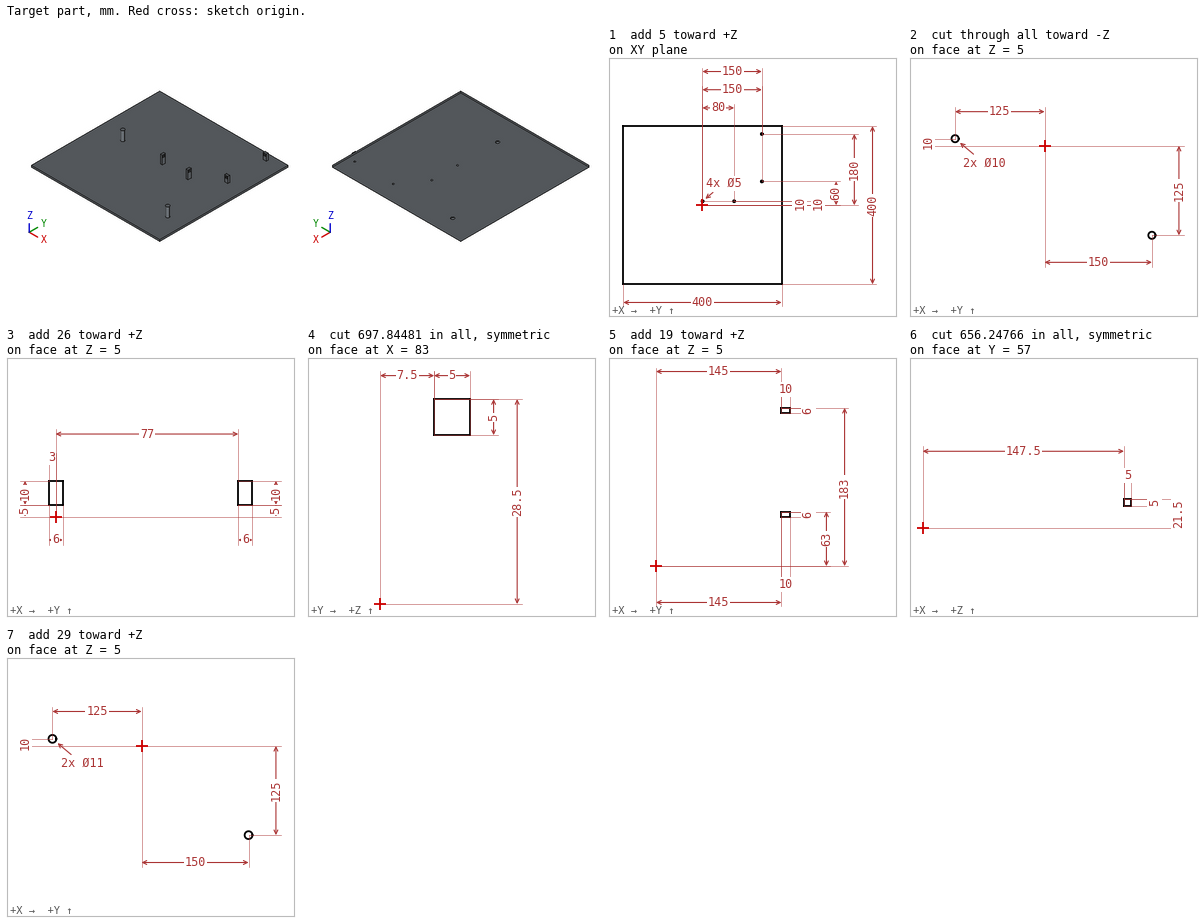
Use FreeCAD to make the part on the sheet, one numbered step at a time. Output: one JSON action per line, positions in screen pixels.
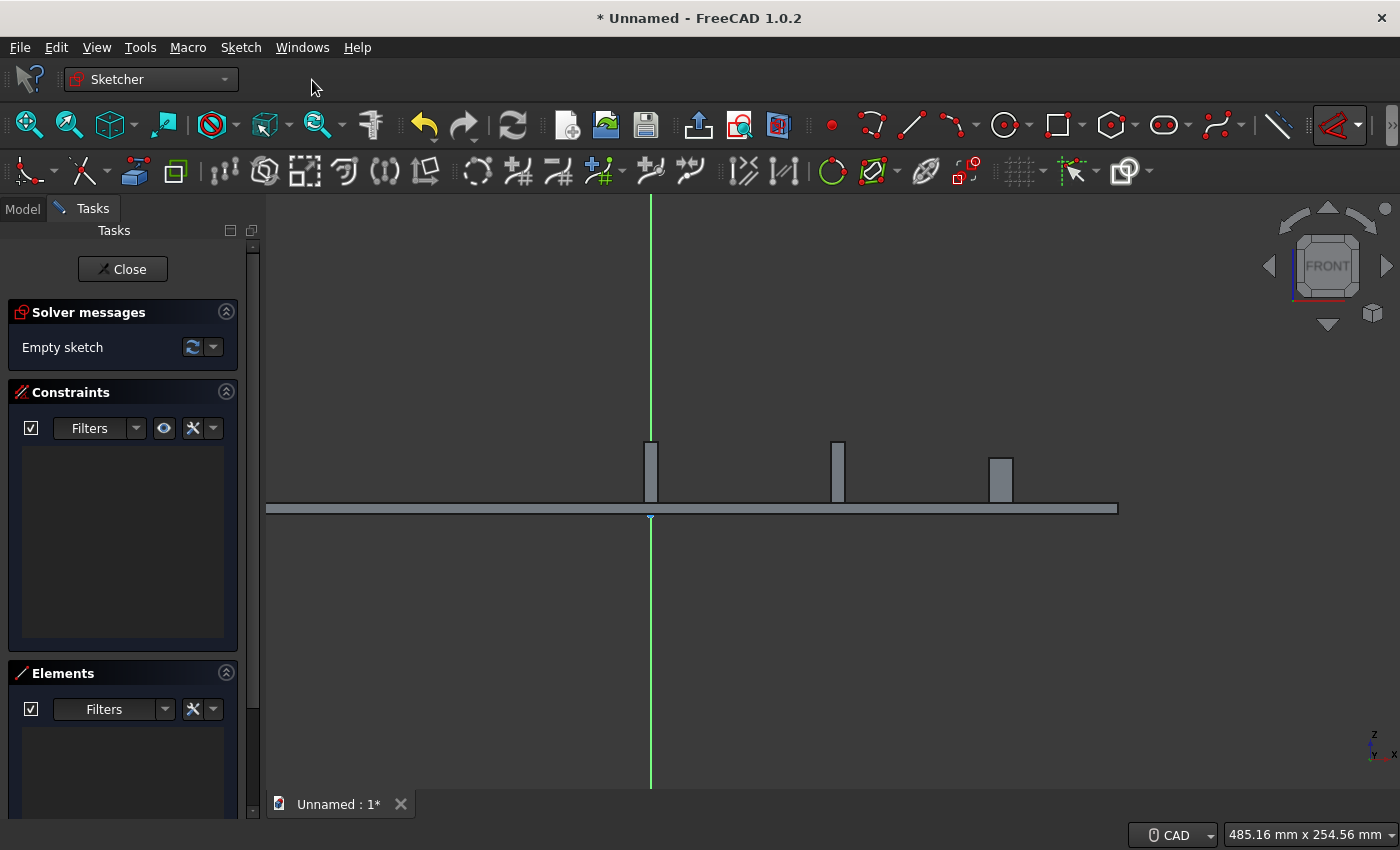
{"action": "scroll", "coordinate": [1014, 469], "scroll_direction": "up", "scroll_amount": 15}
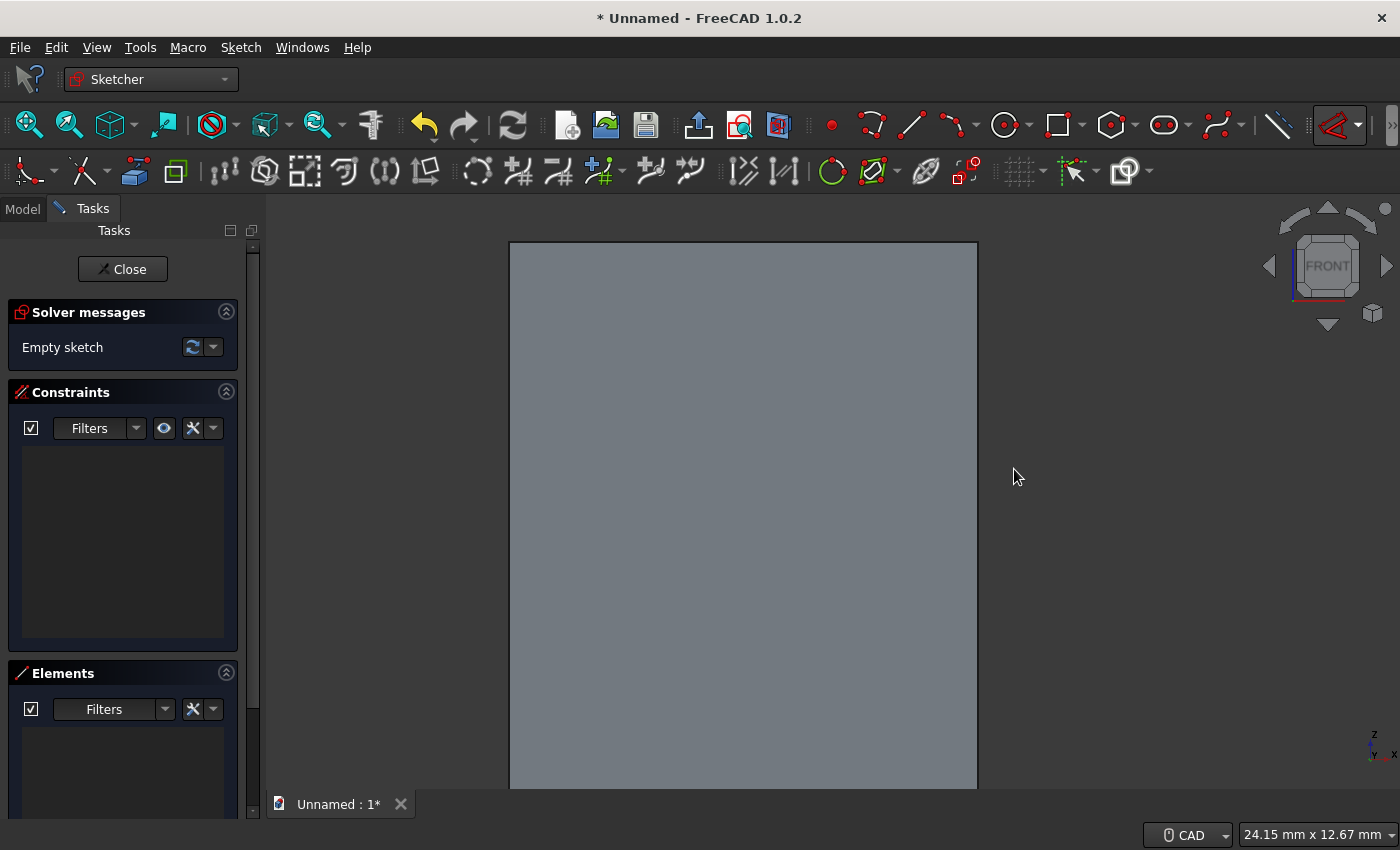
{"action": "scroll", "coordinate": [701, 446], "scroll_direction": "up", "scroll_amount": 2}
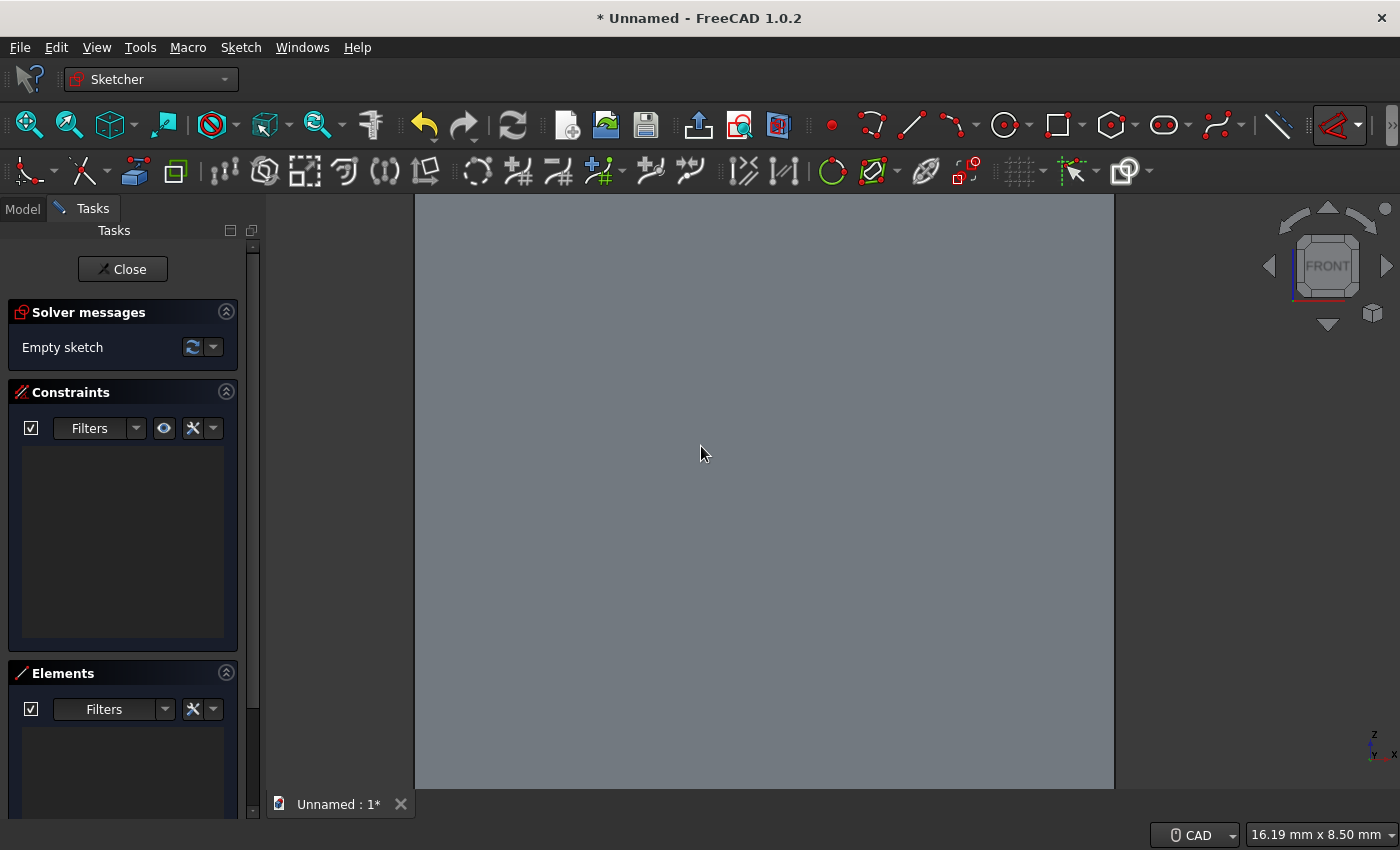
{"action": "key", "text": "g r"}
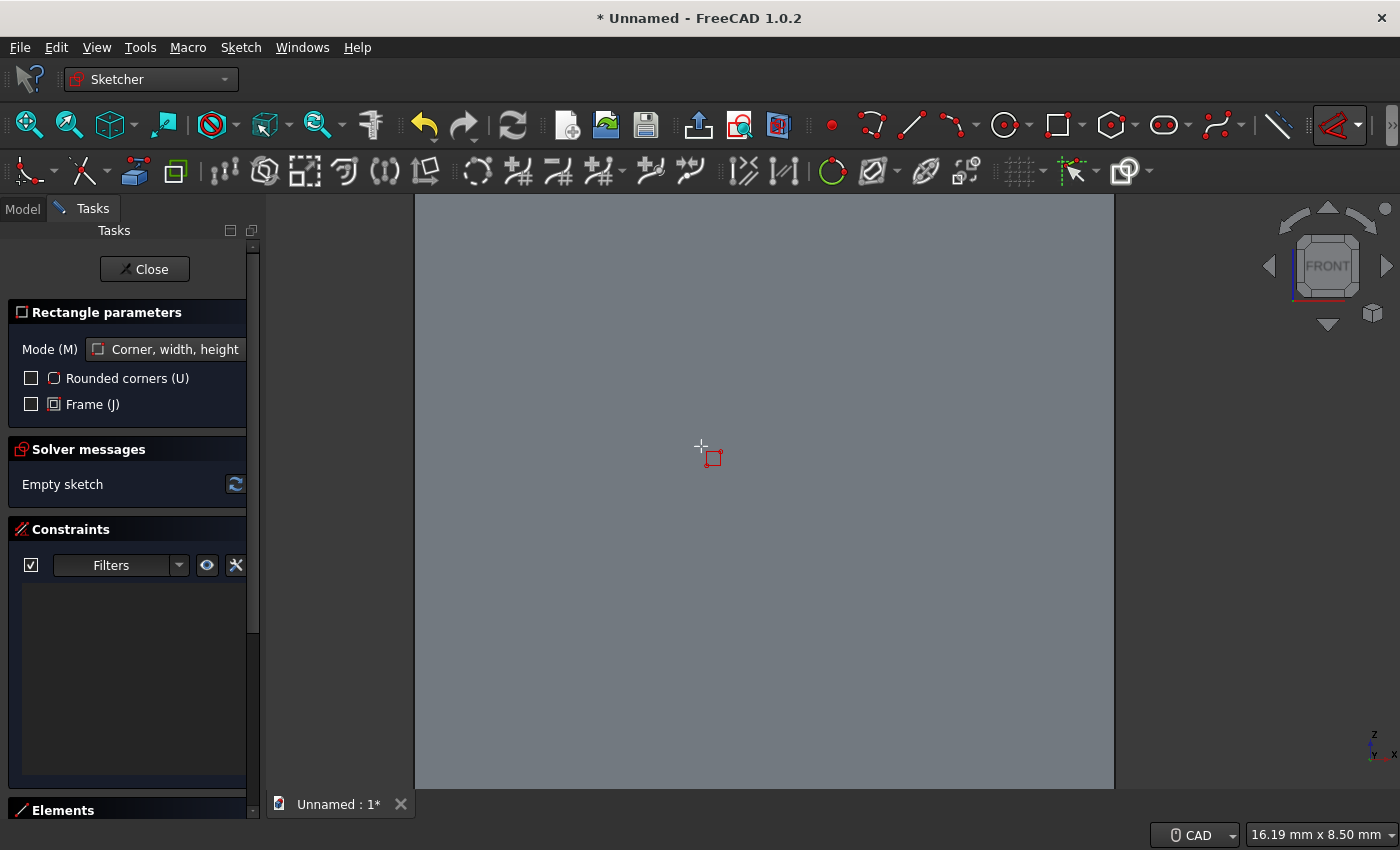
{"action": "left_click", "coordinate": [589, 316]}
{"action": "left_click", "coordinate": [940, 666]}
{"action": "key", "text": "Escape"}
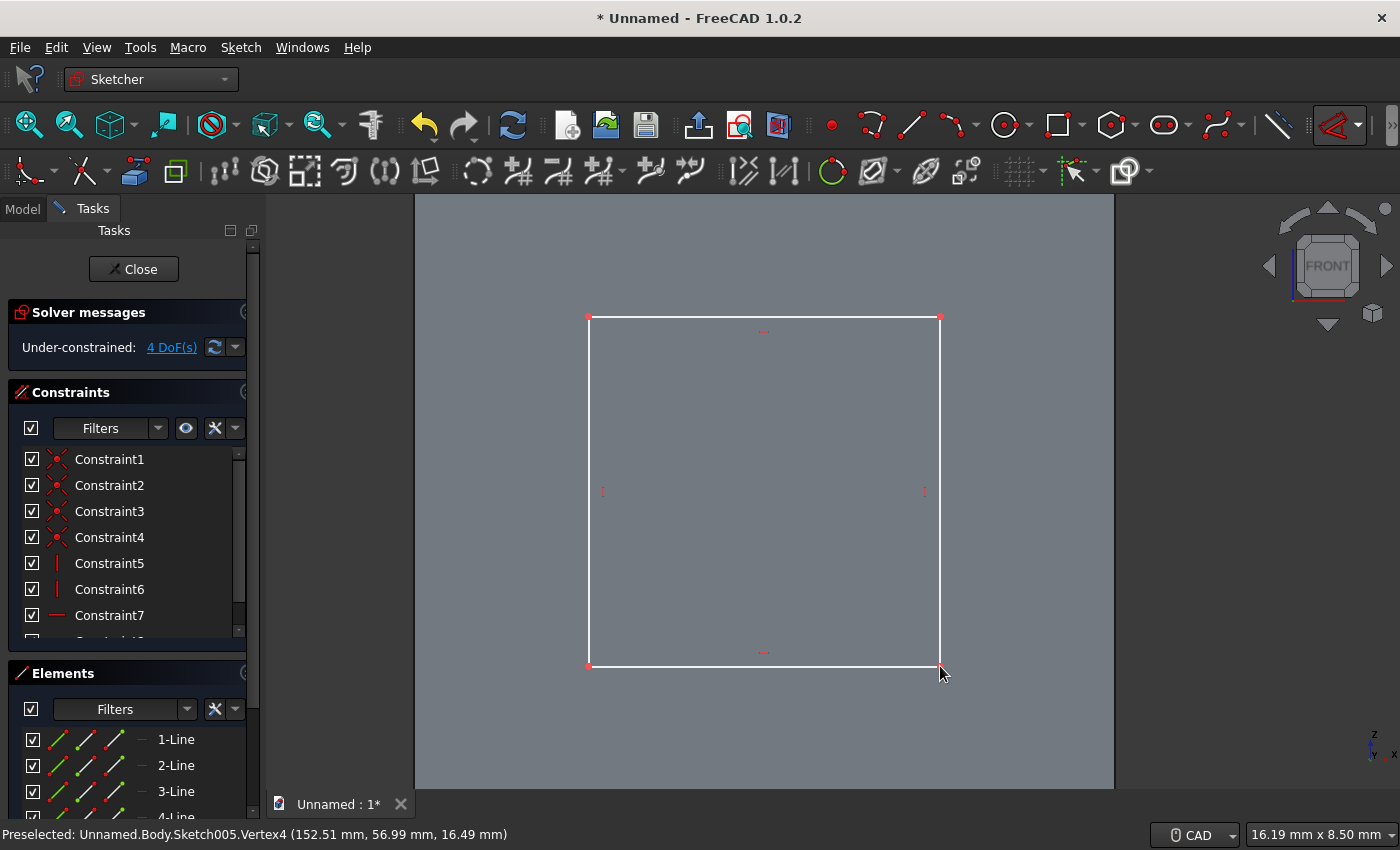
{"action": "left_click", "coordinate": [589, 422]}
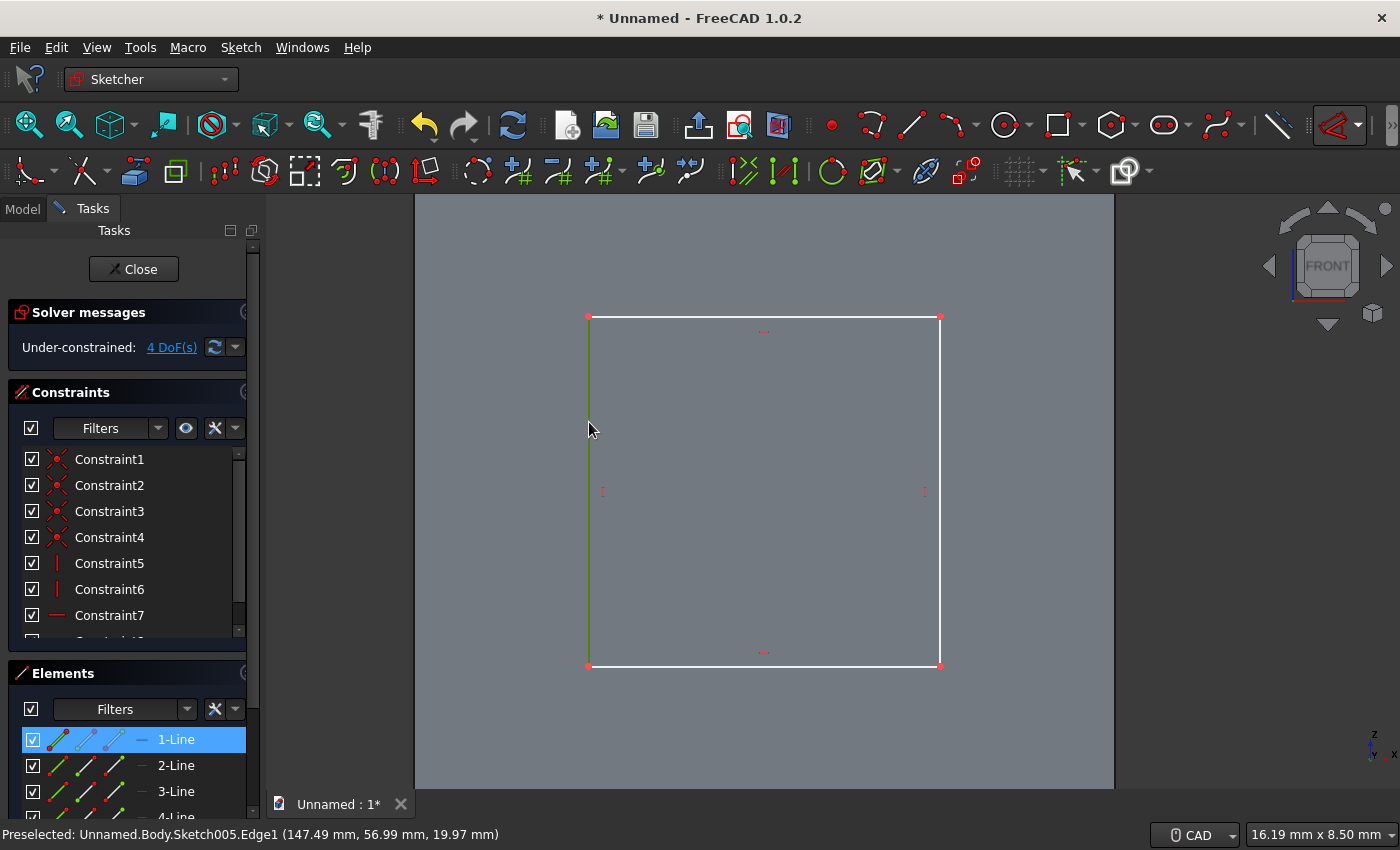
{"action": "key", "text": "i"}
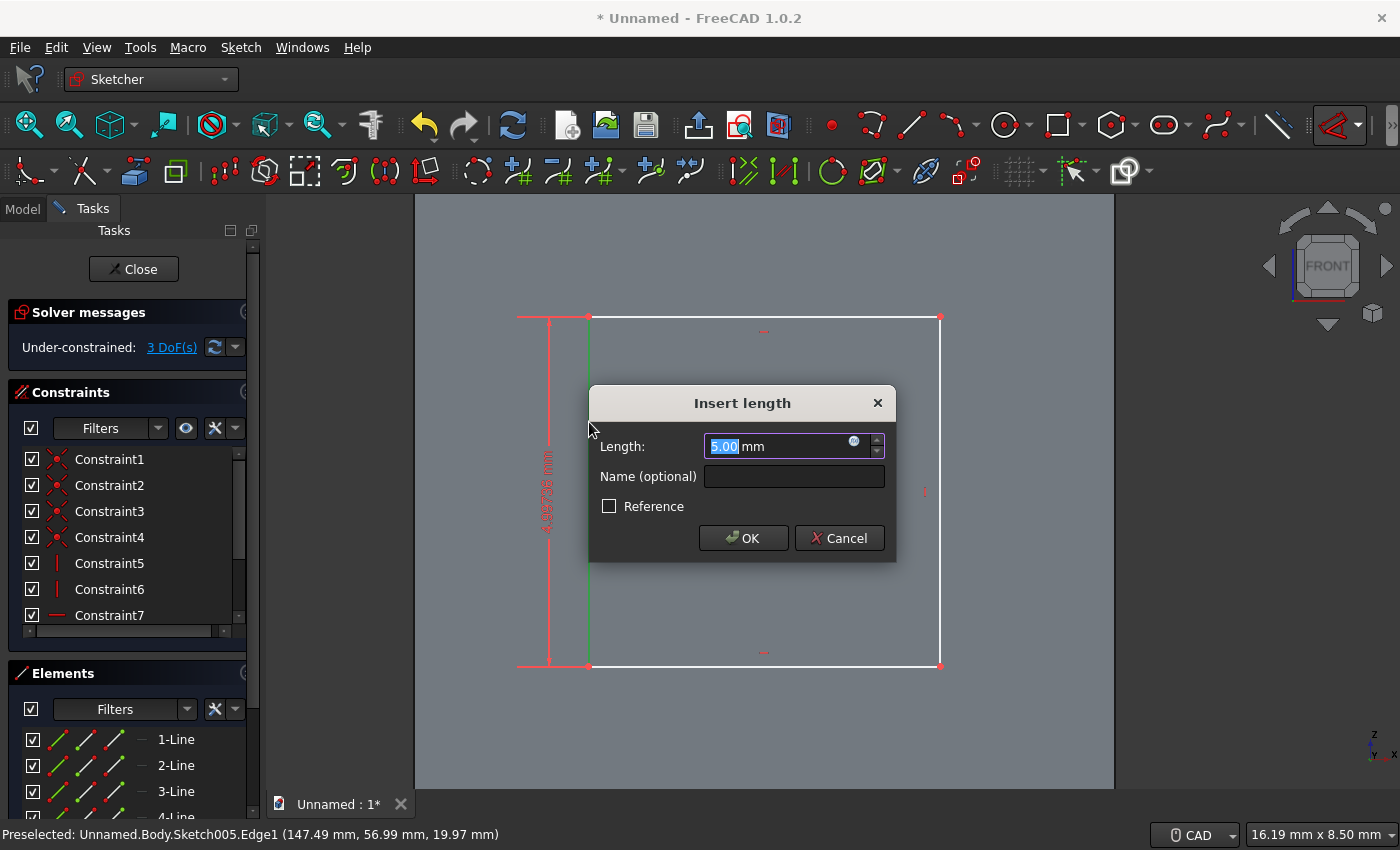
{"action": "type", "text": "5"}
{"action": "key", "text": "Return"}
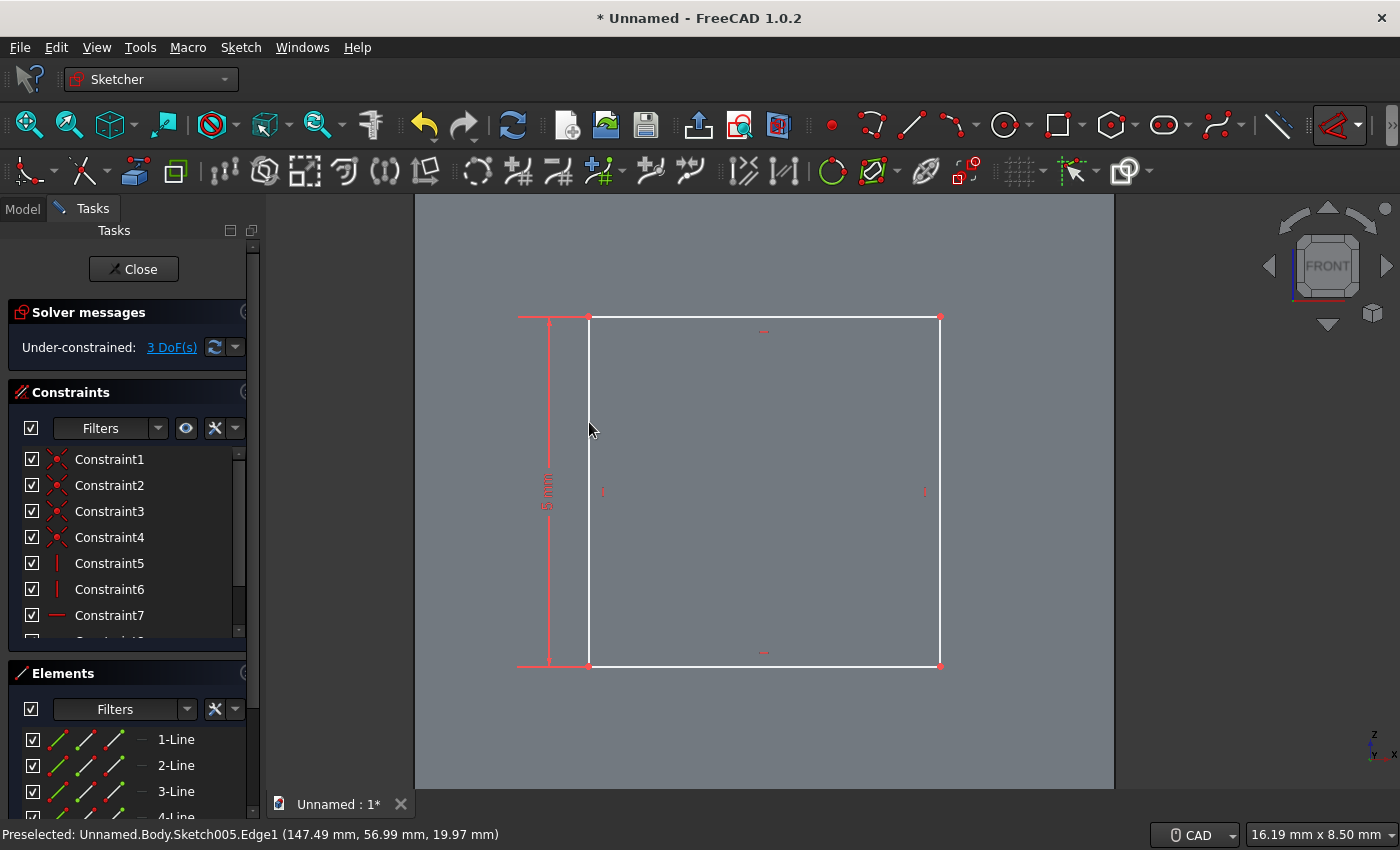
{"action": "left_click", "coordinate": [694, 667]}